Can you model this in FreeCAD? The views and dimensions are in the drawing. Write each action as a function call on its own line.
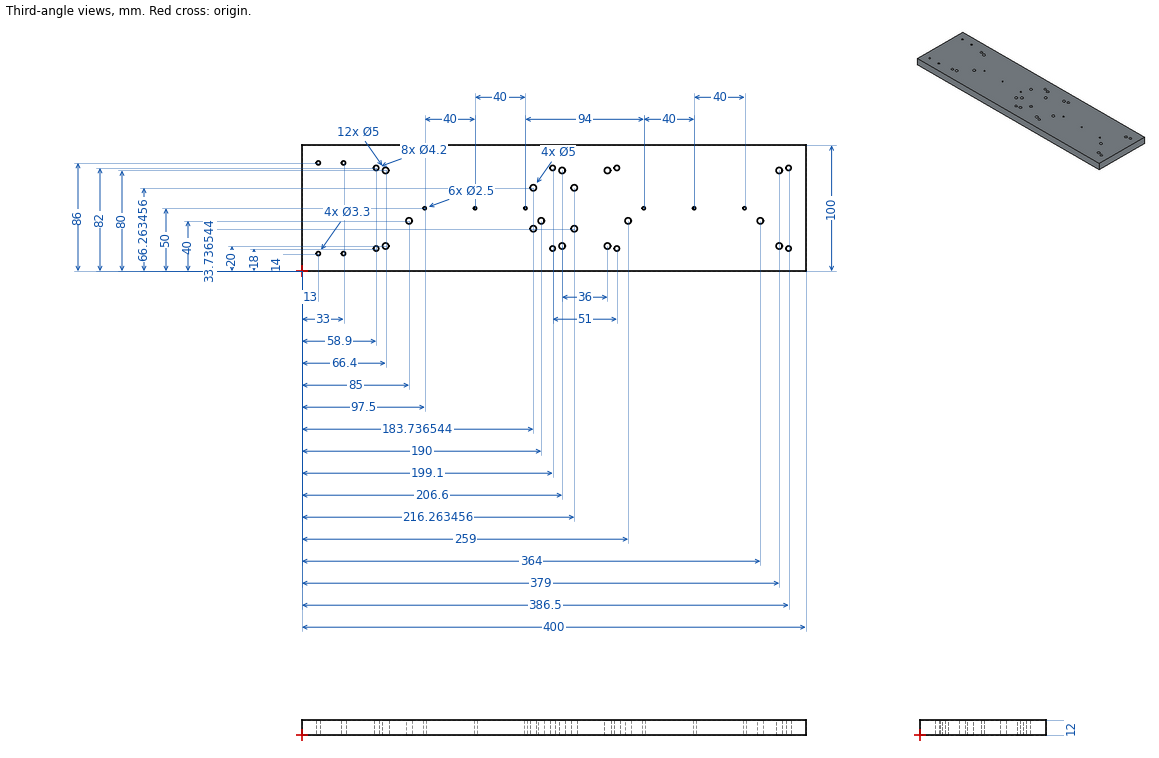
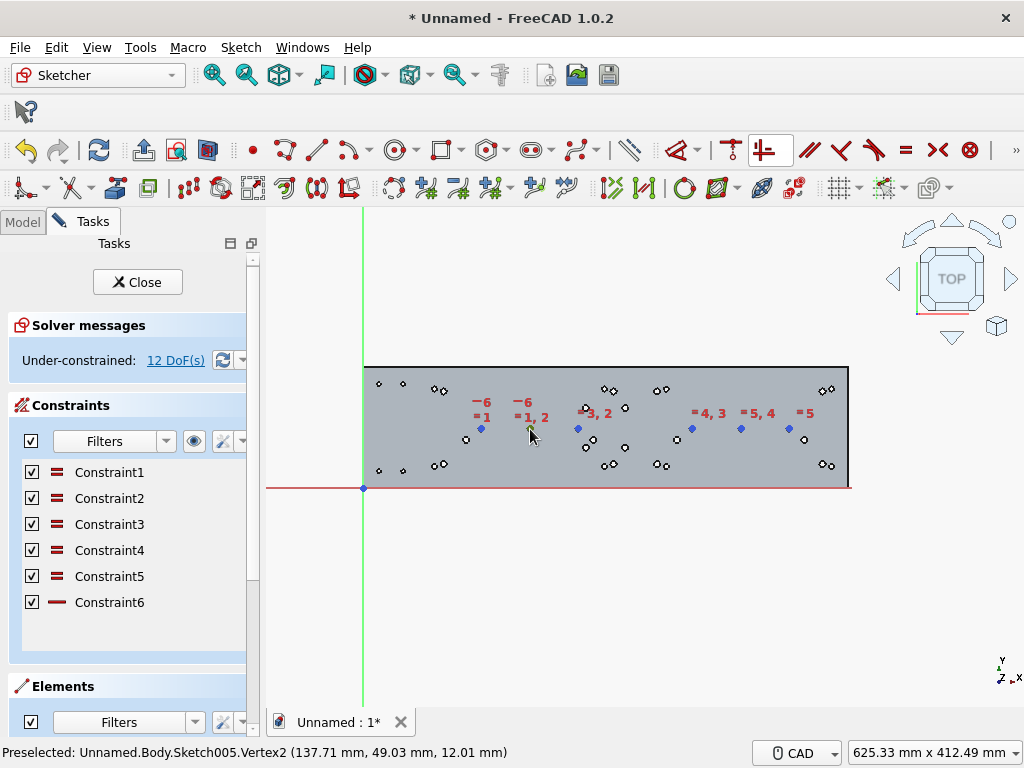
click(578, 429)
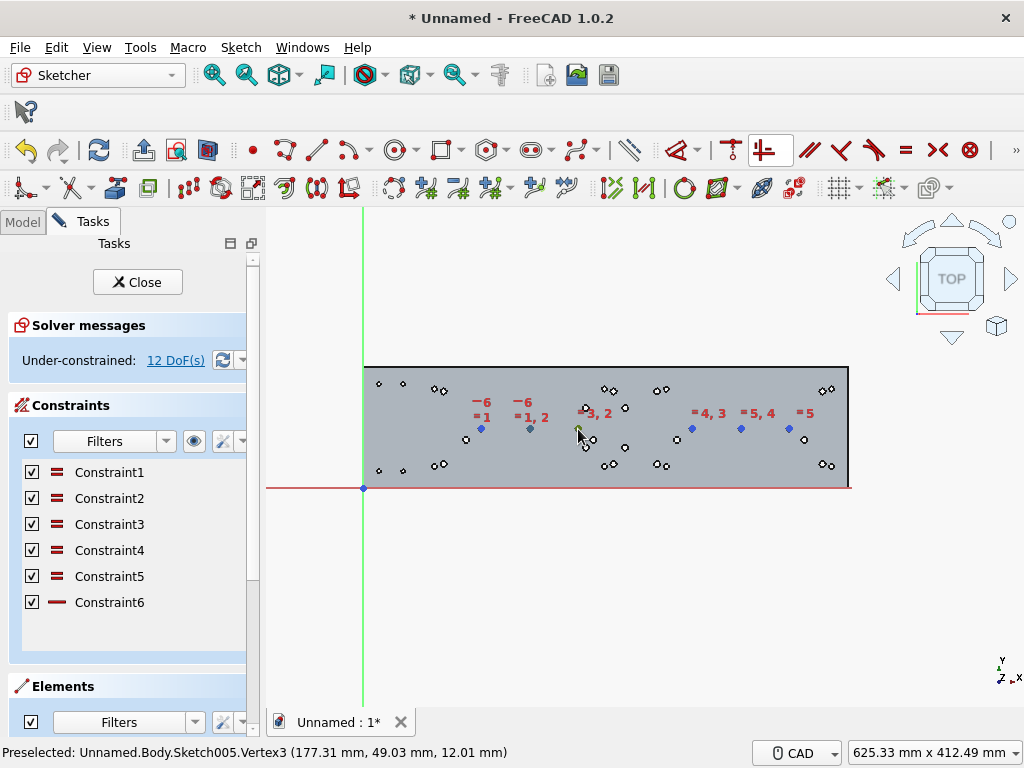
click(788, 150)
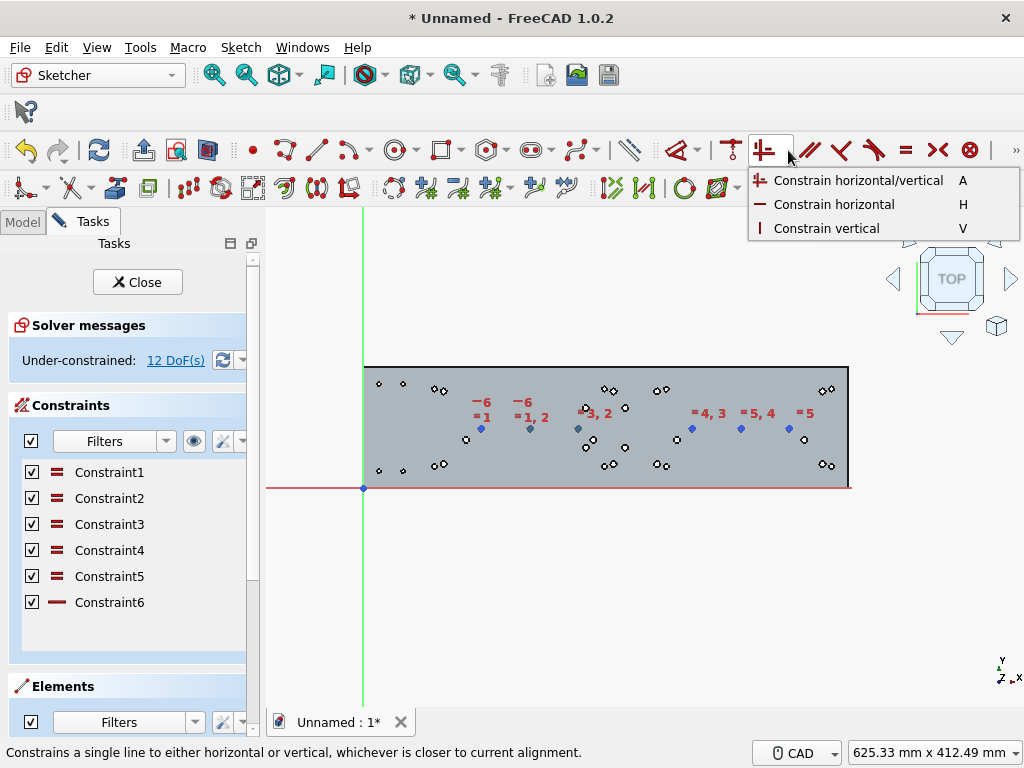
click(884, 204)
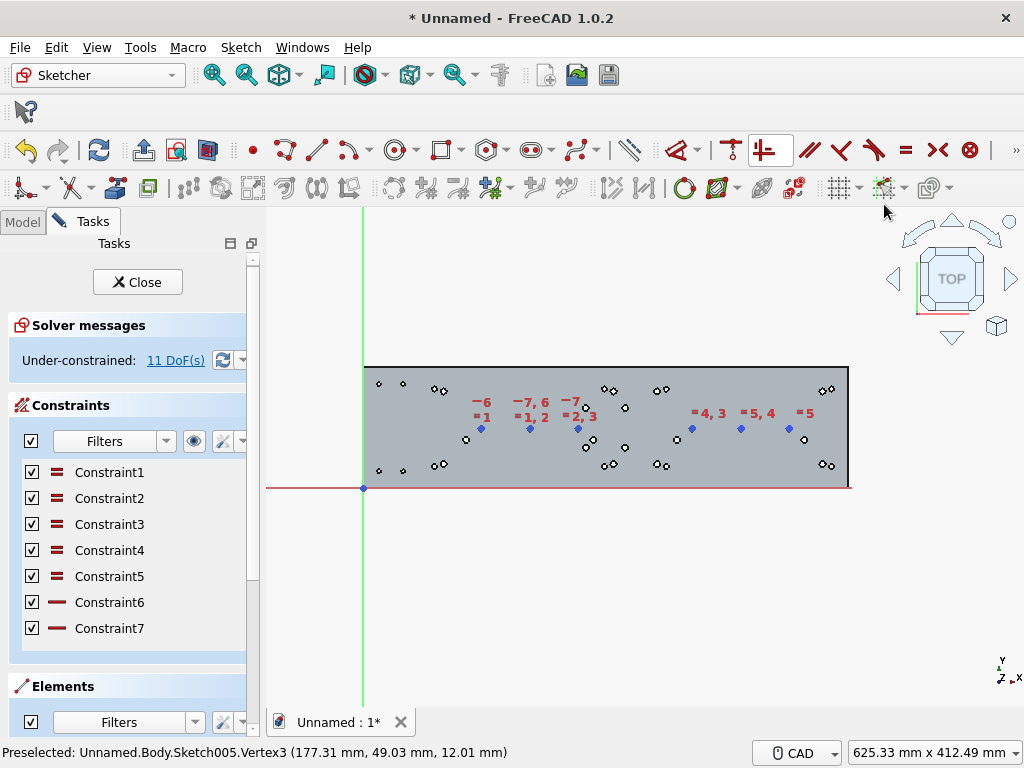
click(578, 429)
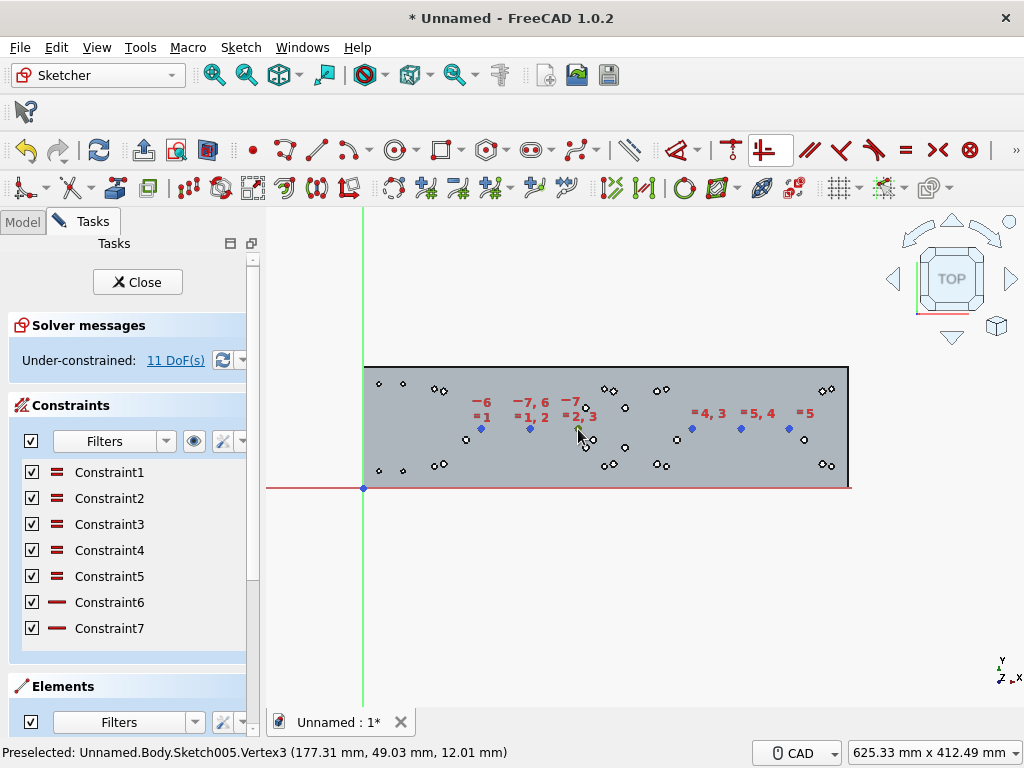
click(692, 429)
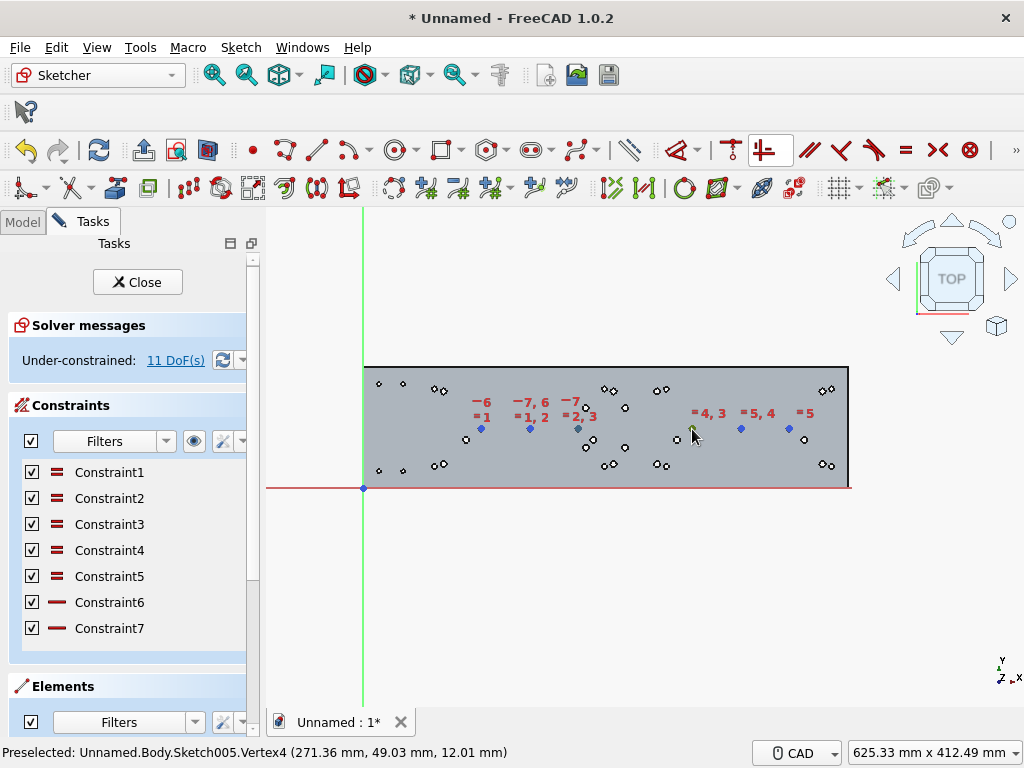
click(788, 150)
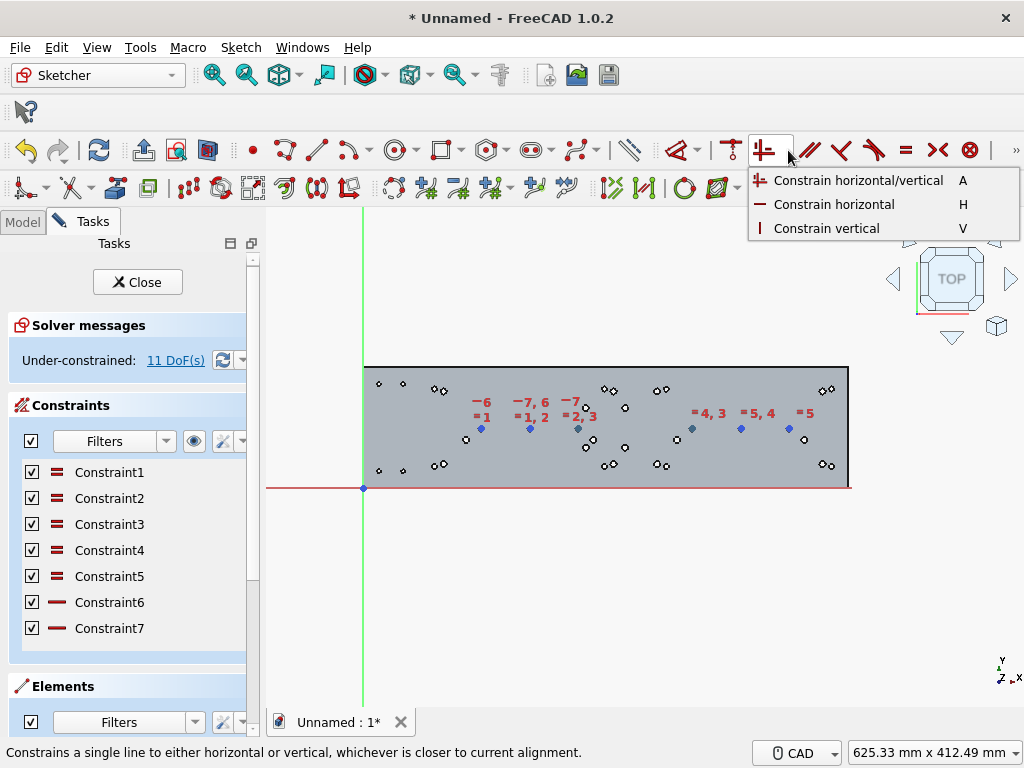
click(884, 204)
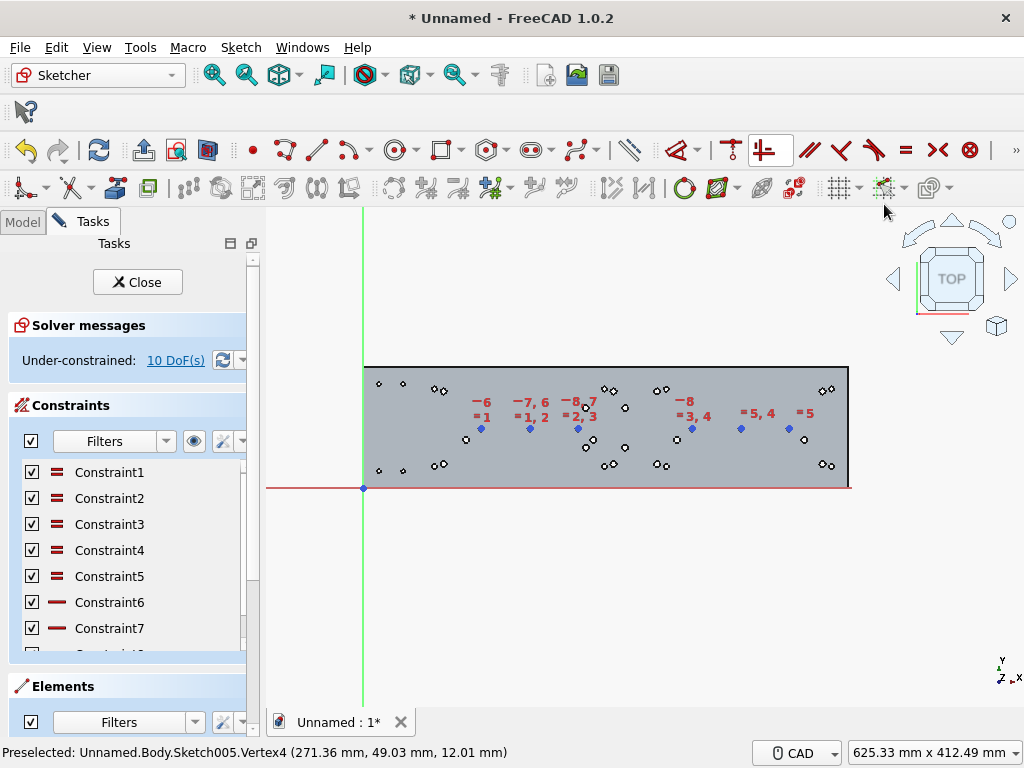
click(692, 429)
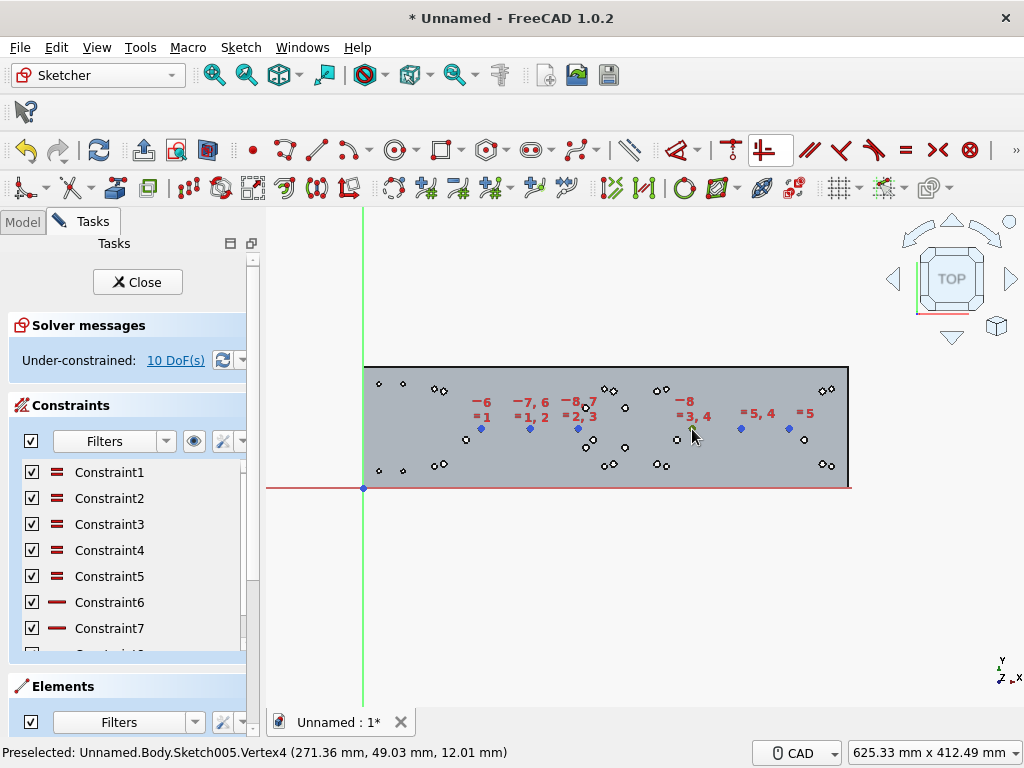
click(741, 429)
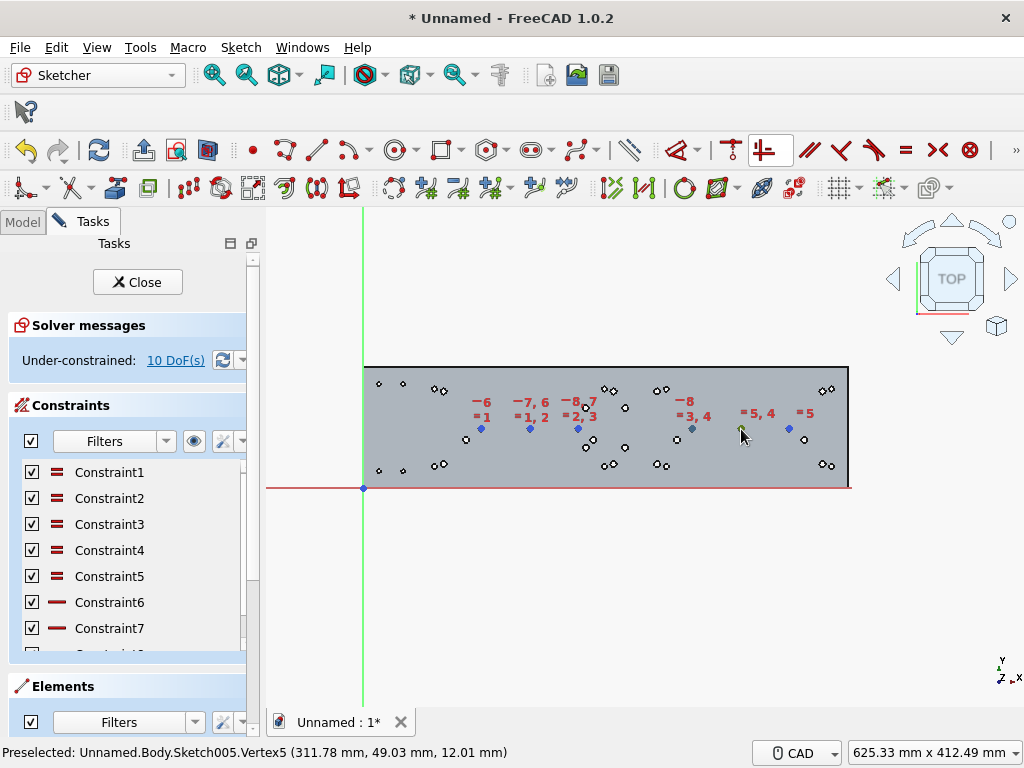
click(788, 150)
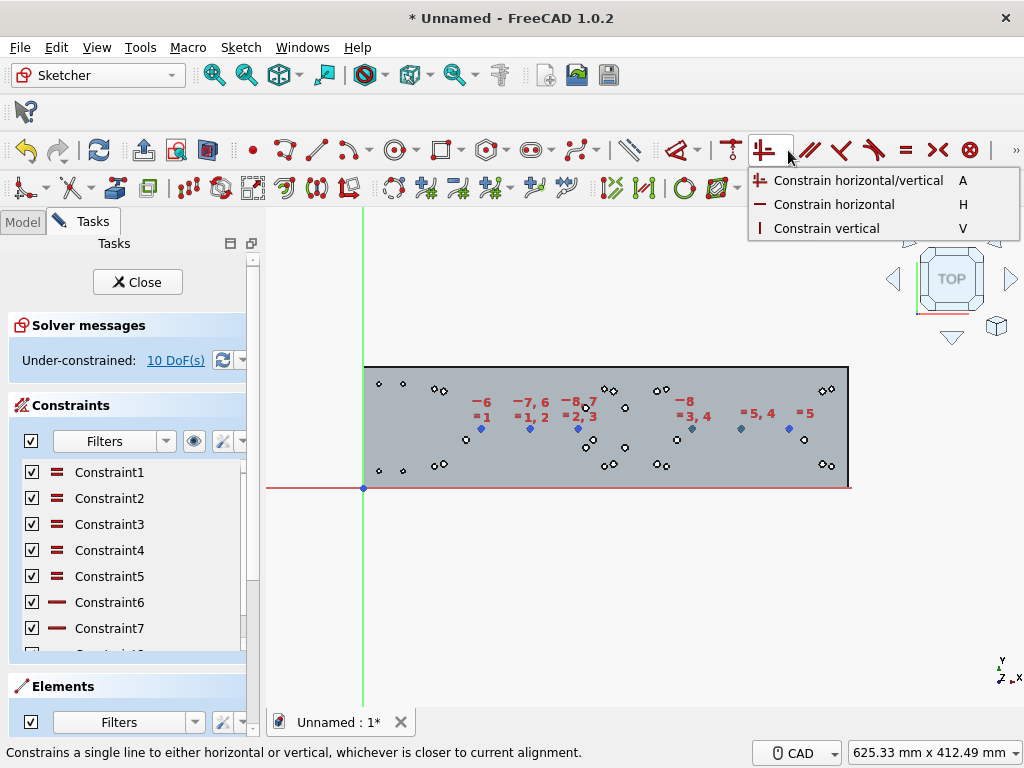
click(884, 204)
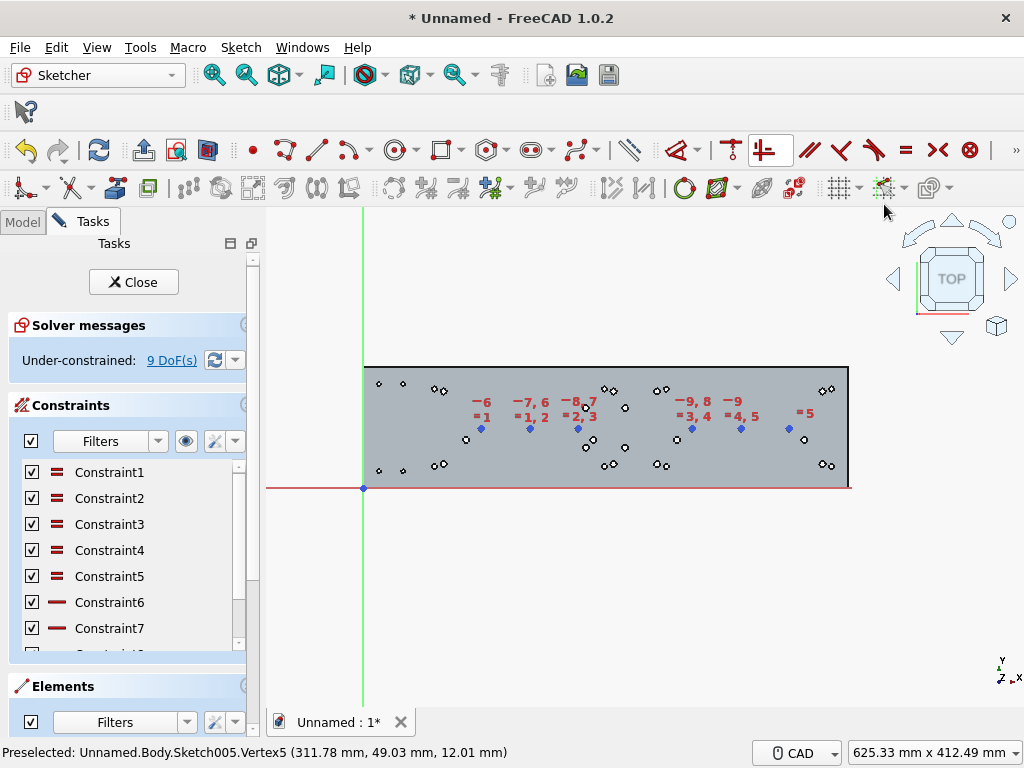
click(741, 429)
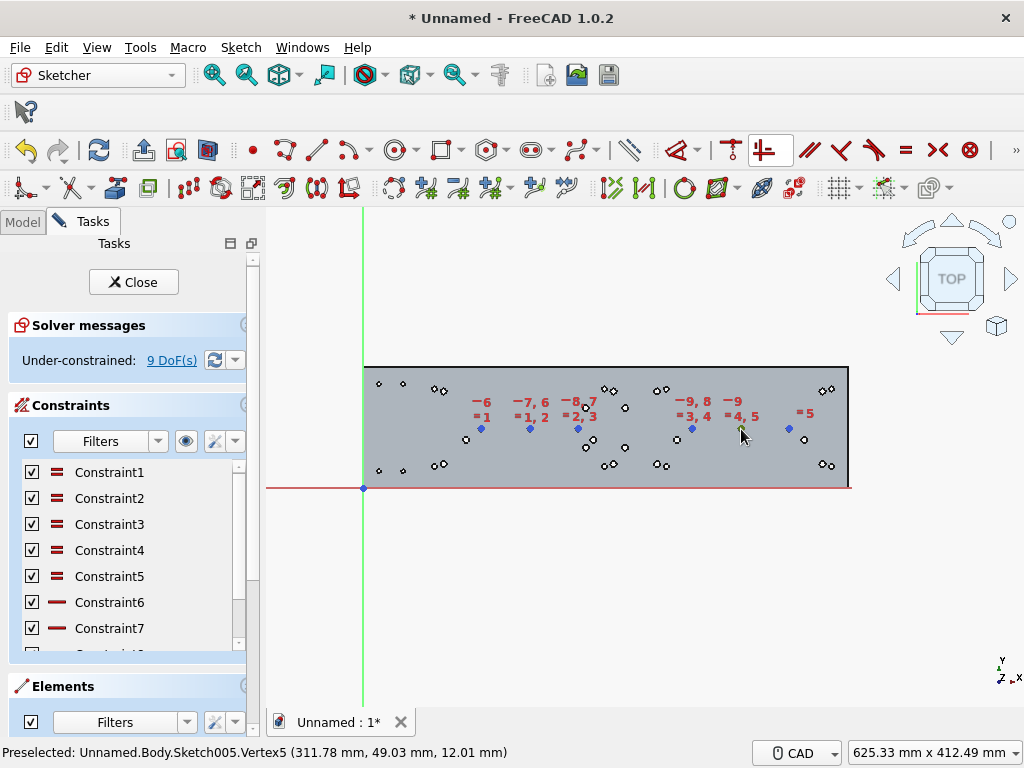
click(789, 429)